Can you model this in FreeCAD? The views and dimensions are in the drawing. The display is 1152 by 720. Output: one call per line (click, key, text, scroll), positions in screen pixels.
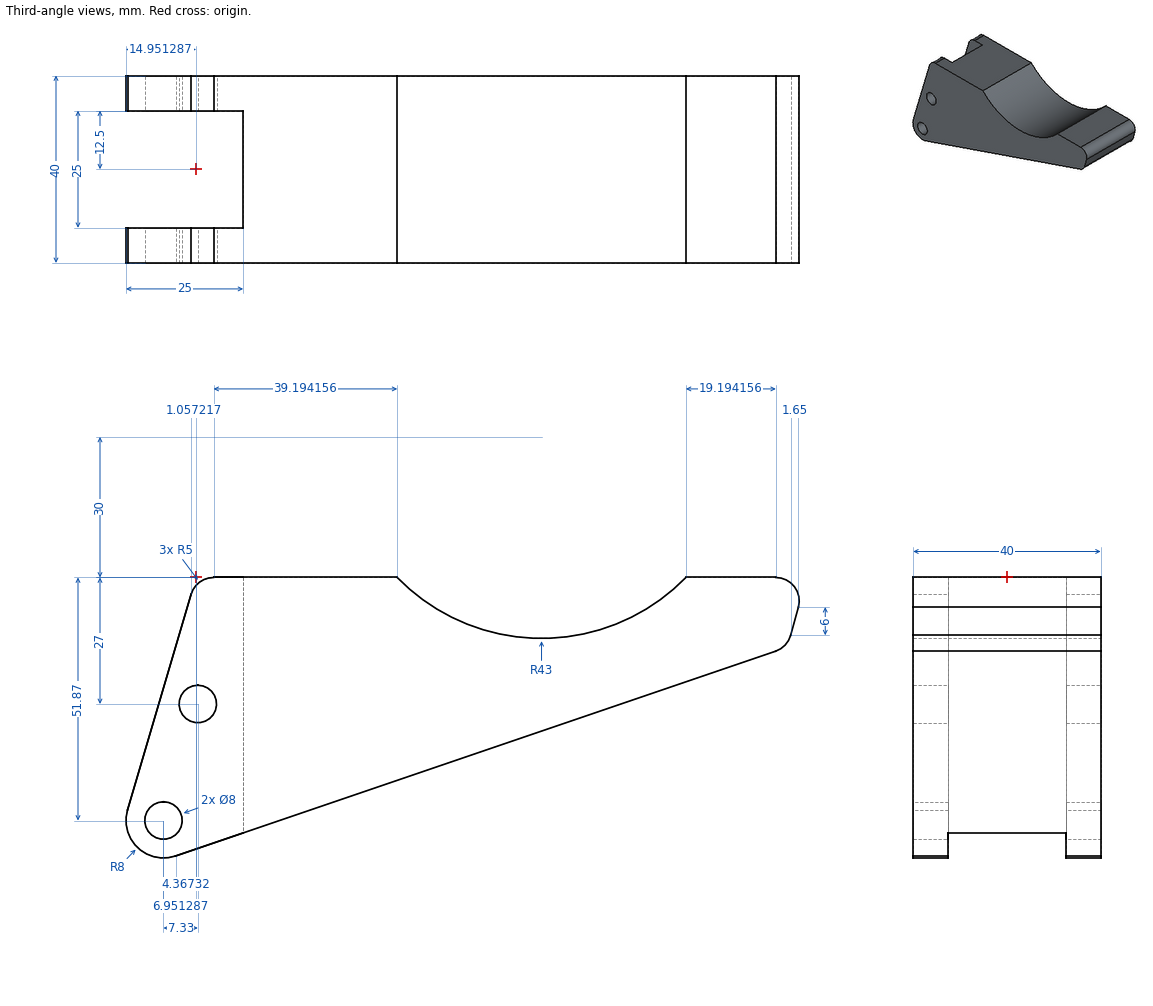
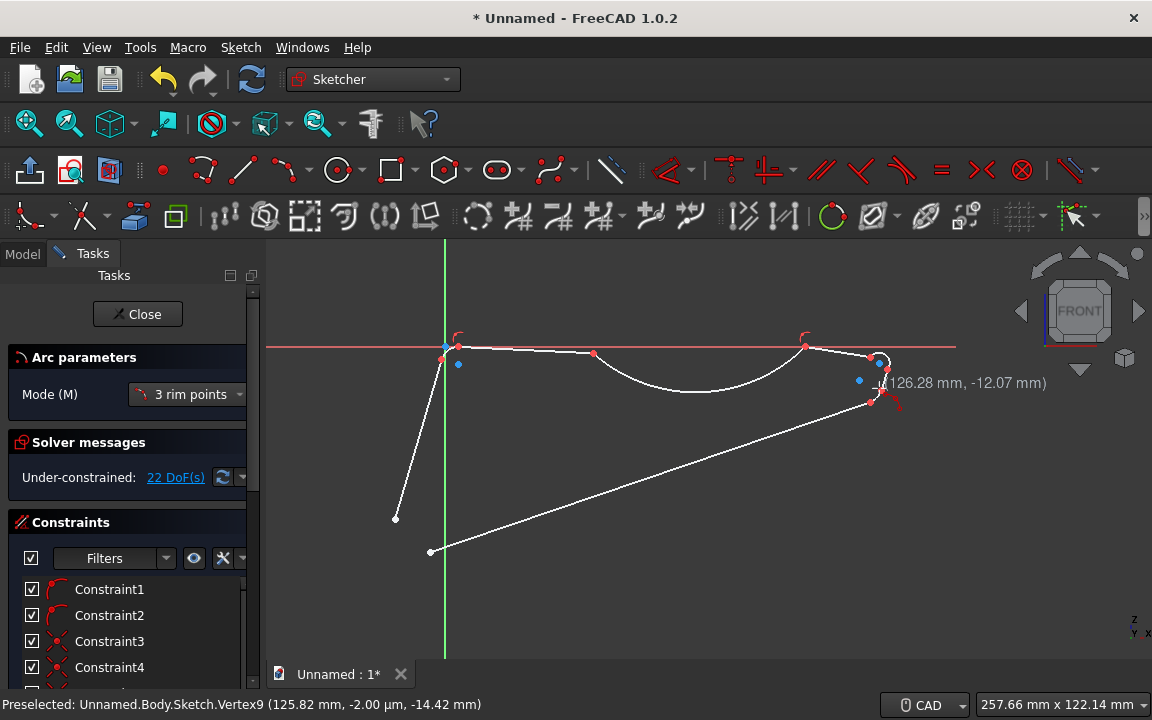
click(431, 552)
click(395, 519)
click(402, 545)
key(Escape)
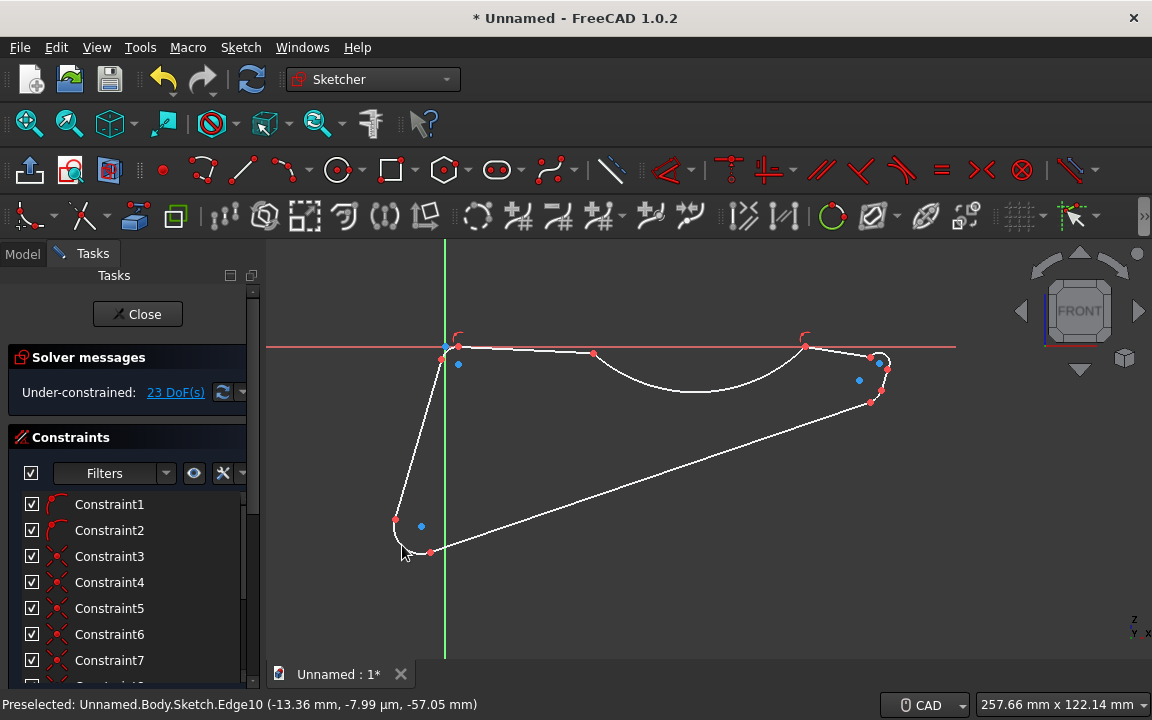
click(409, 471)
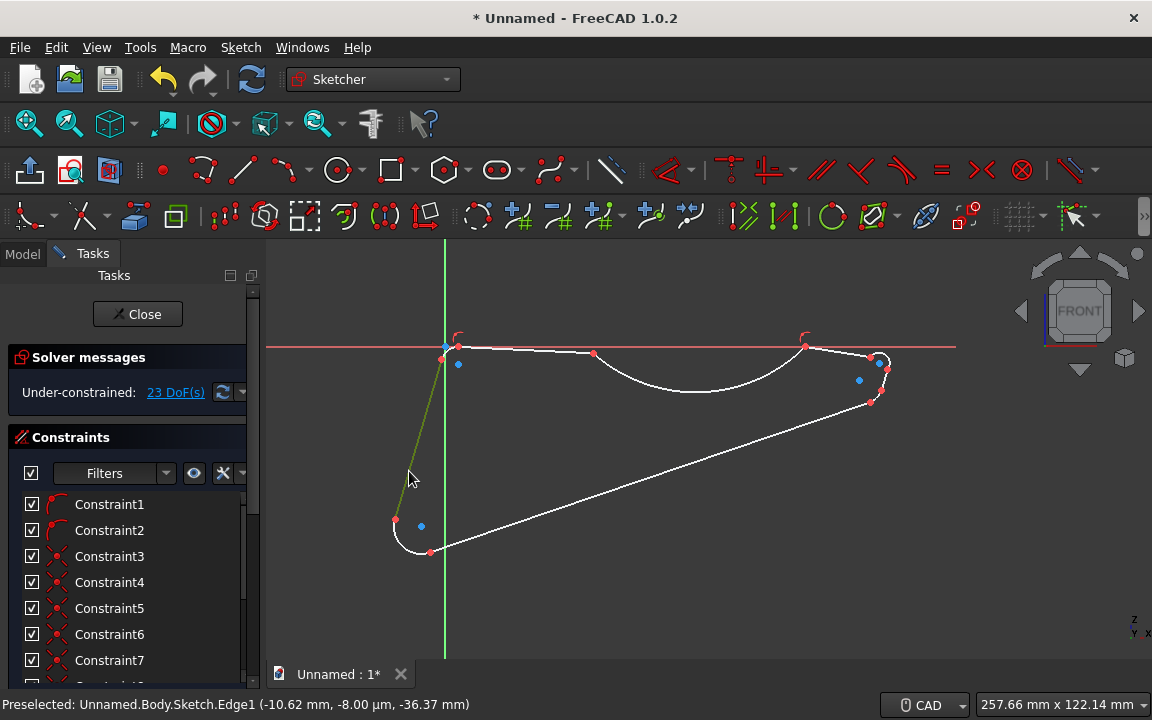
scroll(448, 350, up, 2)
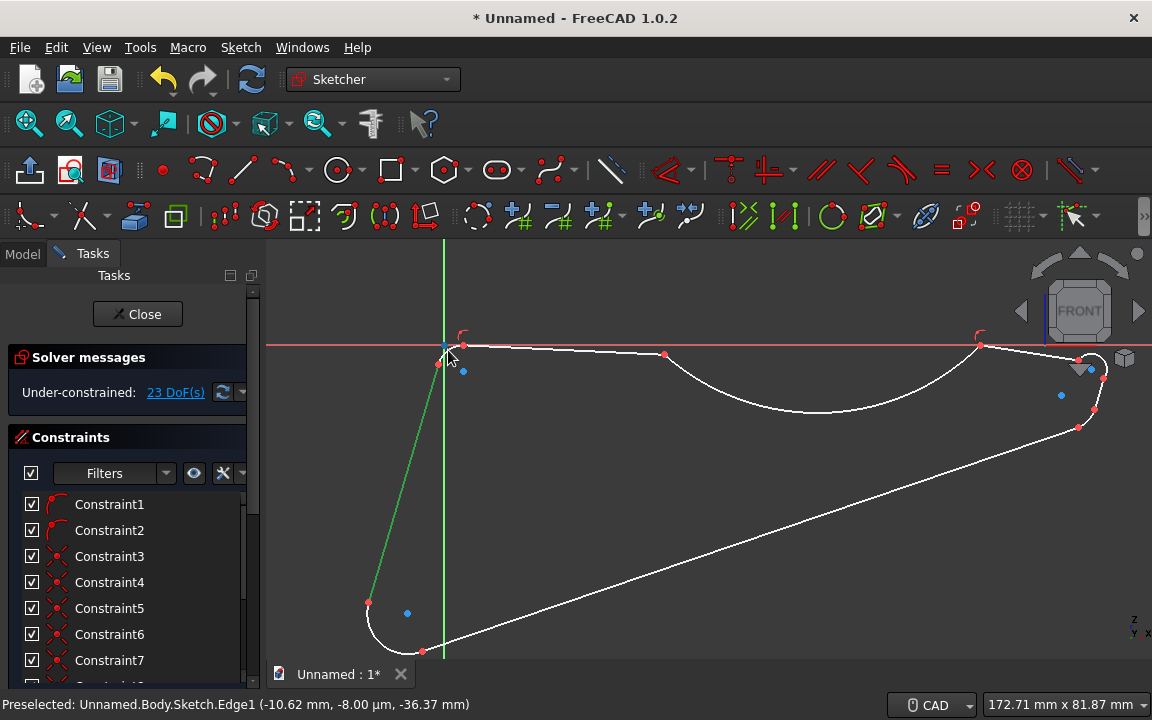
click(448, 350)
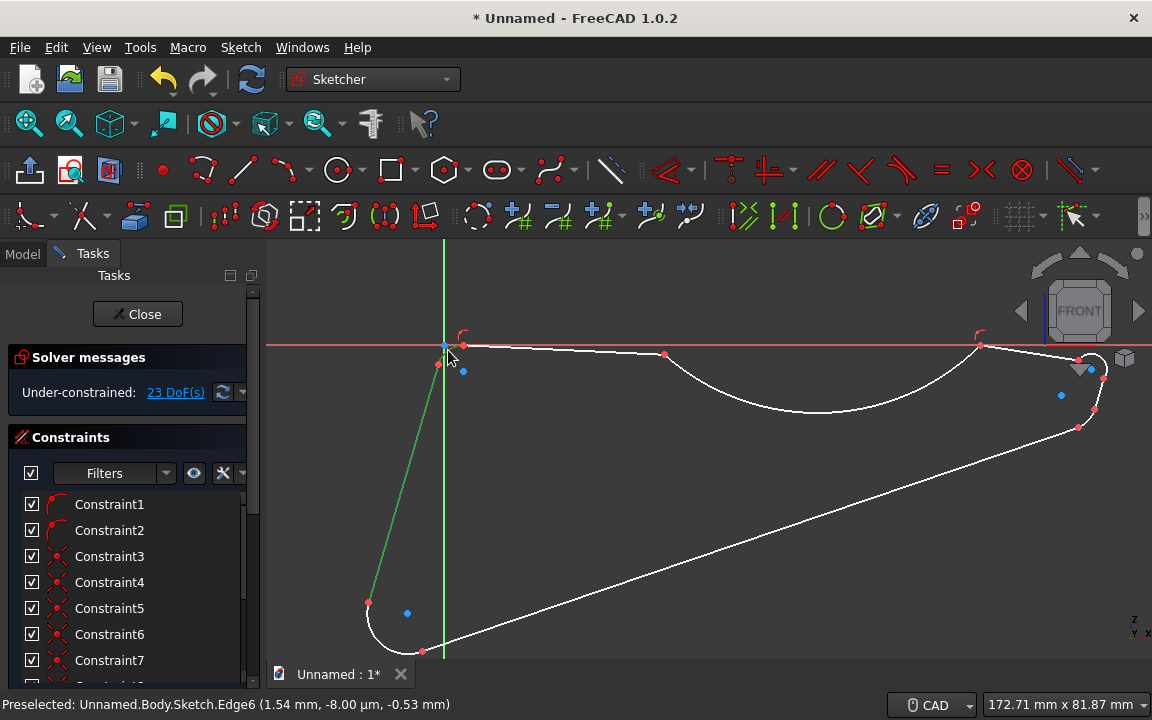
click(902, 170)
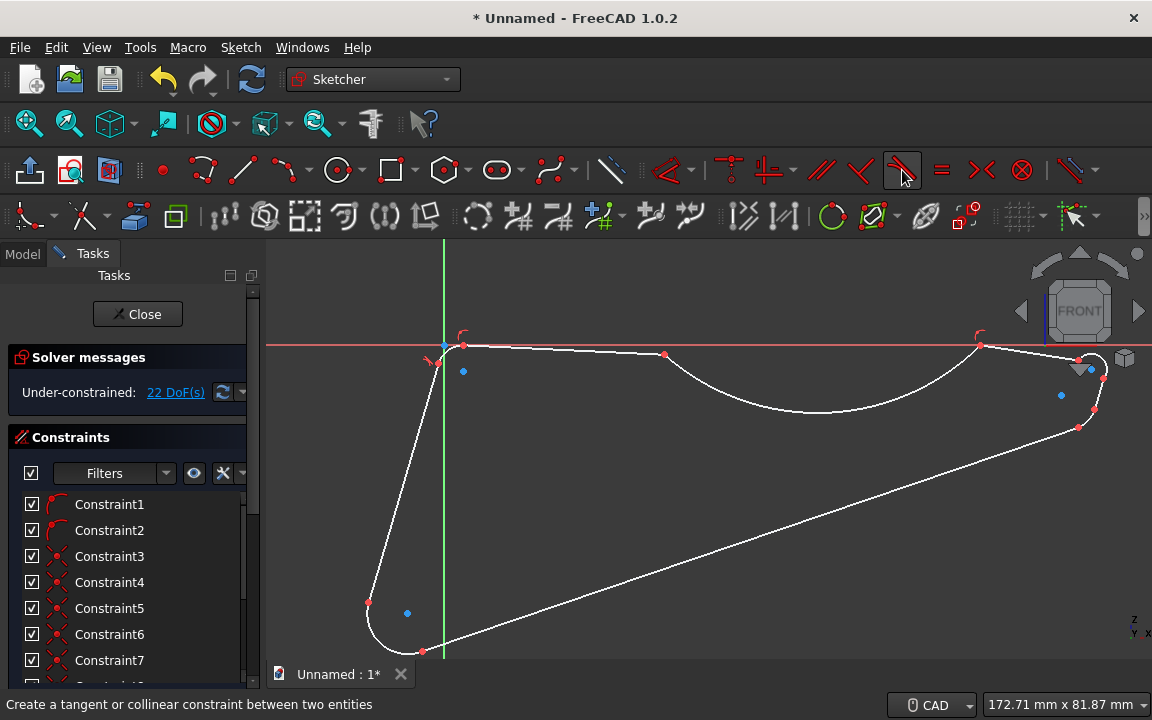
click(390, 531)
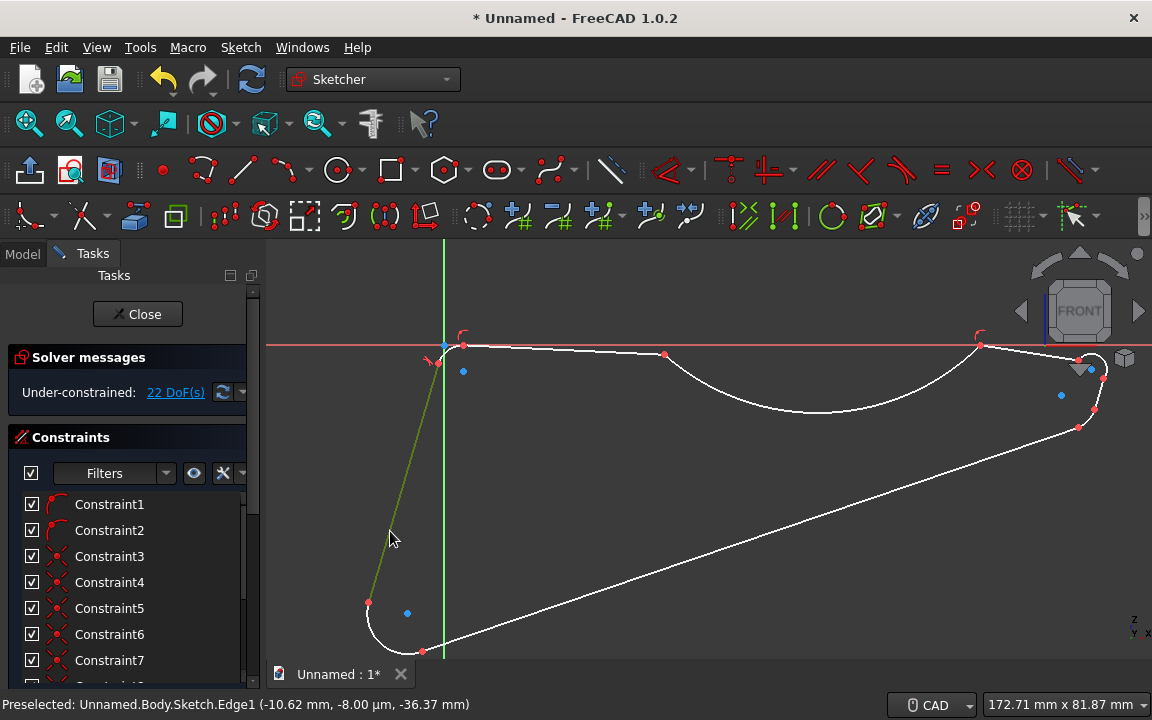
click(370, 629)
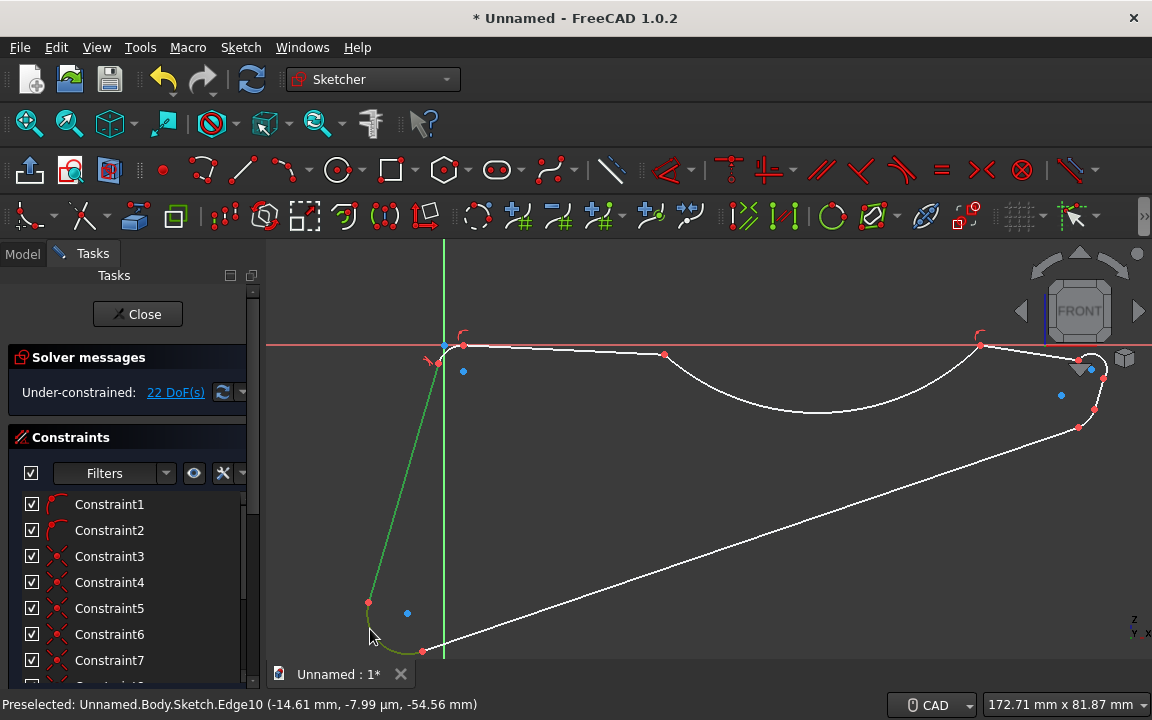
key(t)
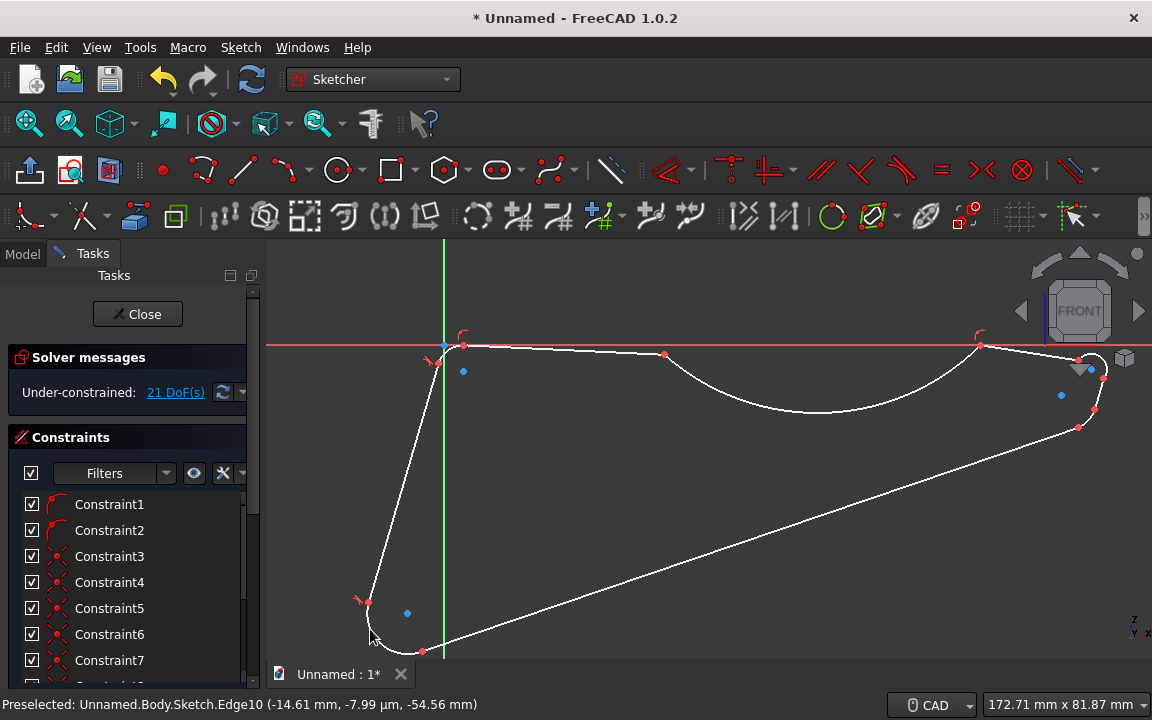
click(524, 348)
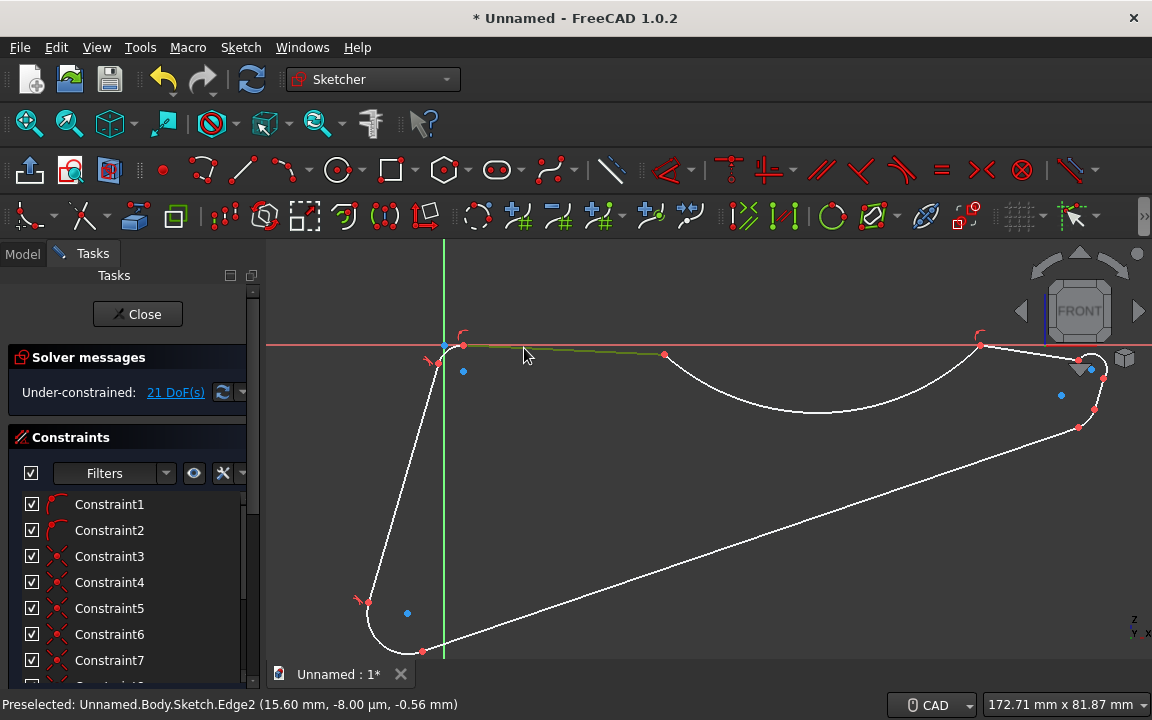
scroll(454, 347, up, 2)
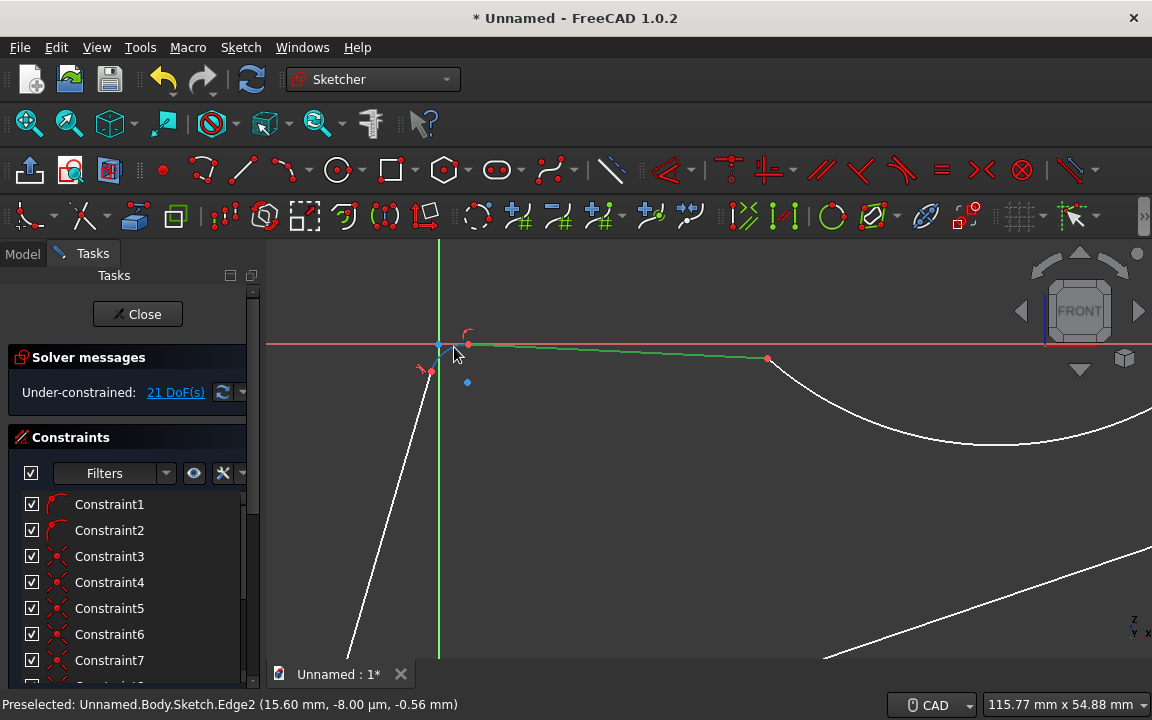
click(454, 347)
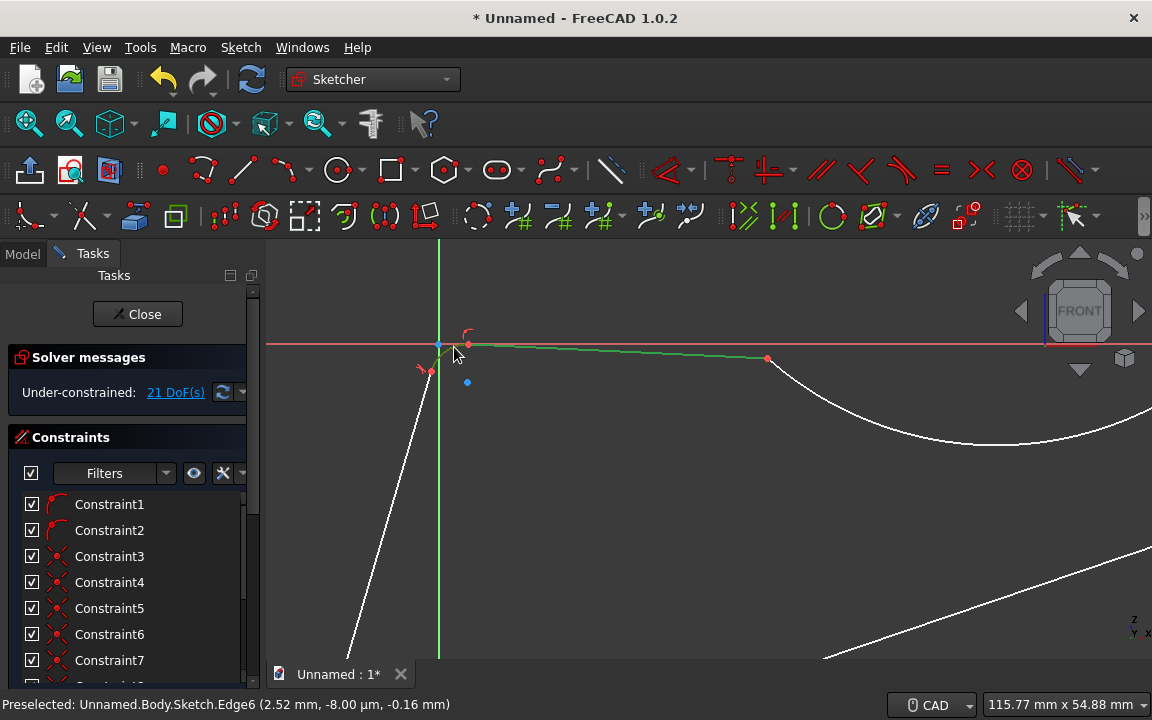
click(902, 170)